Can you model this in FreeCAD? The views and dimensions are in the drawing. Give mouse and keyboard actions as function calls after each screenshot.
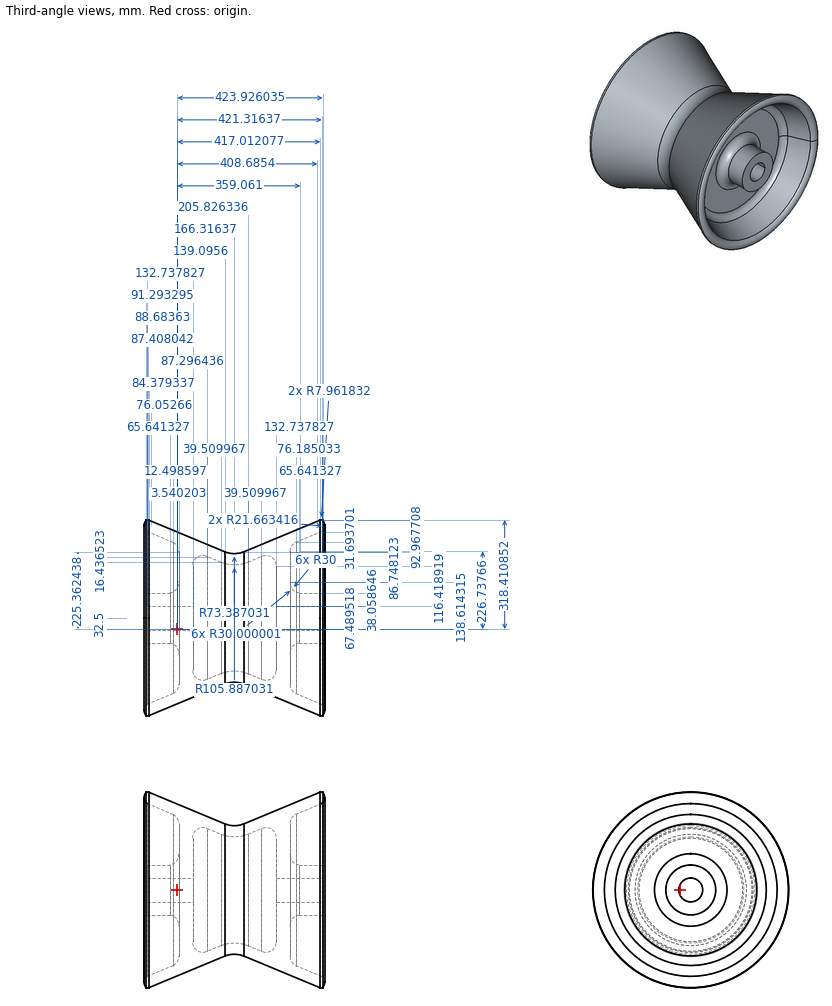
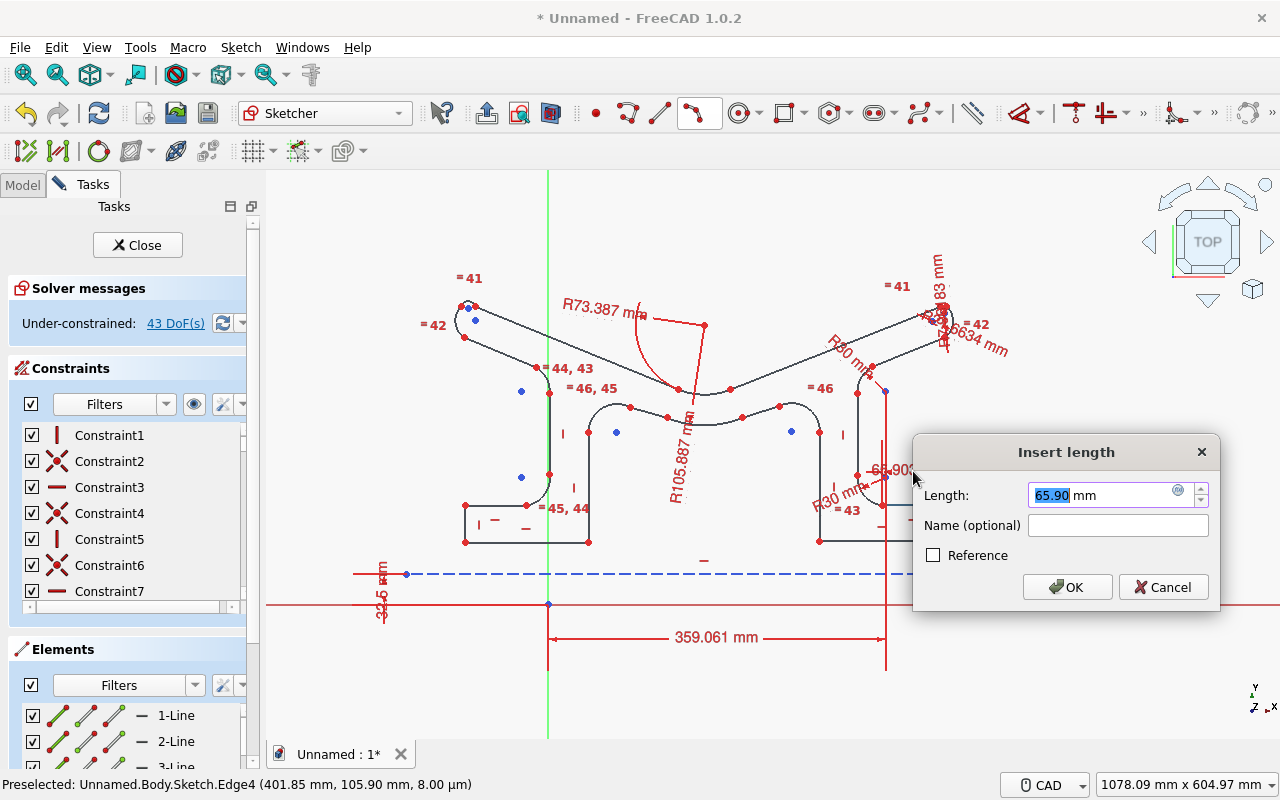
text(65.641327)
key(Return)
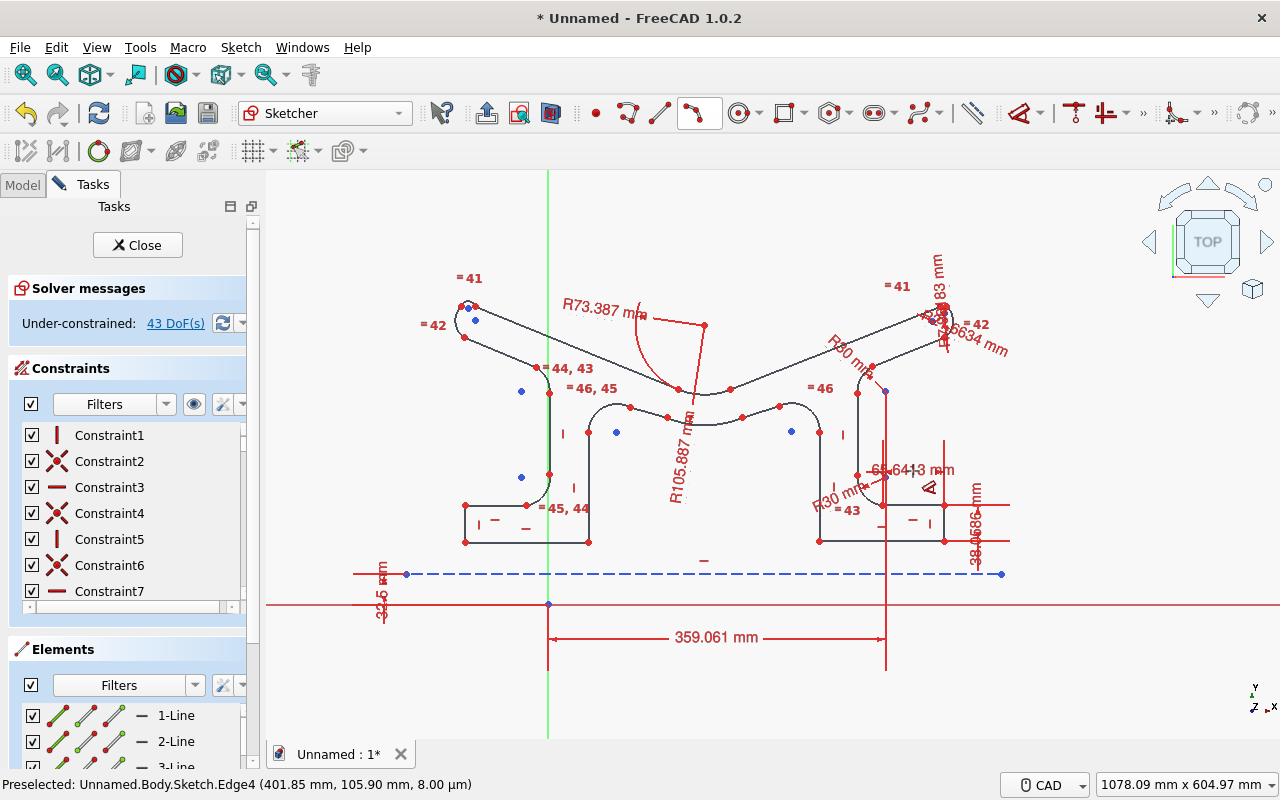
click(858, 451)
click(892, 435)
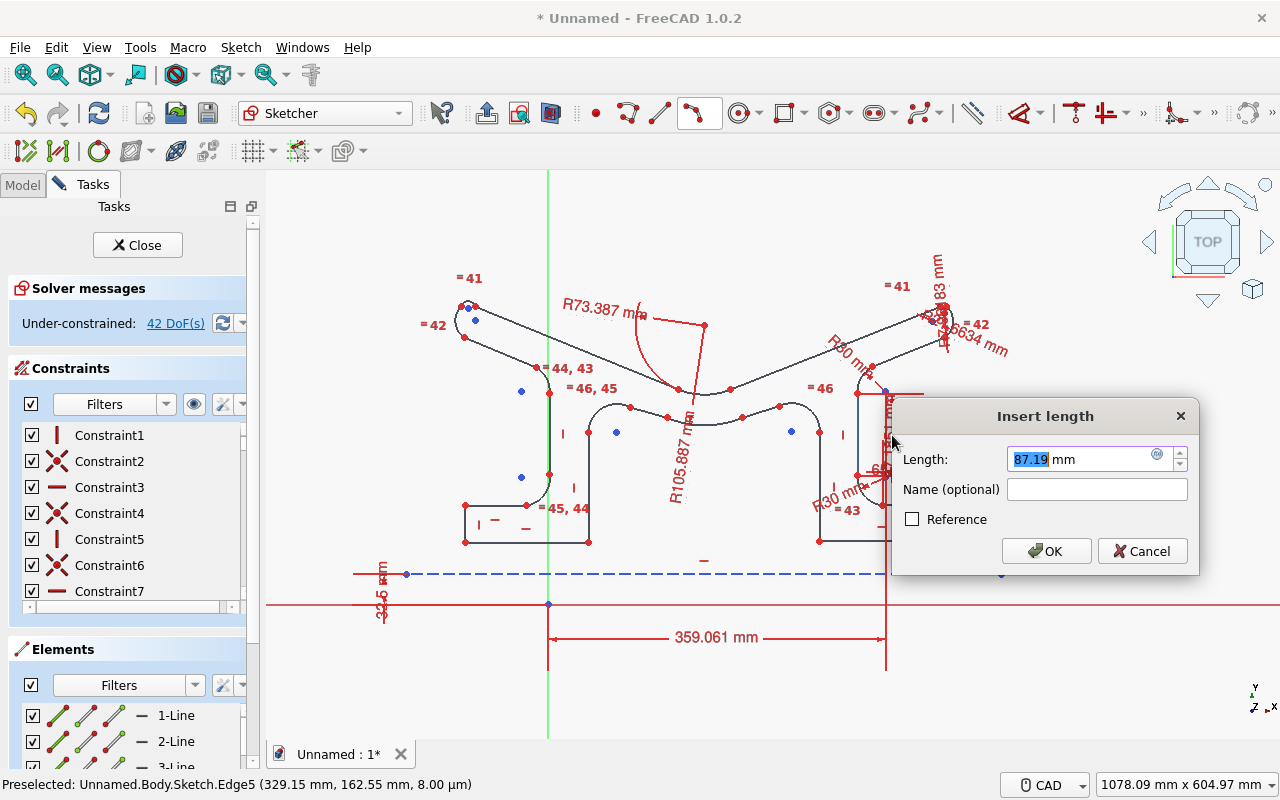
text(86.748123)
key(Return)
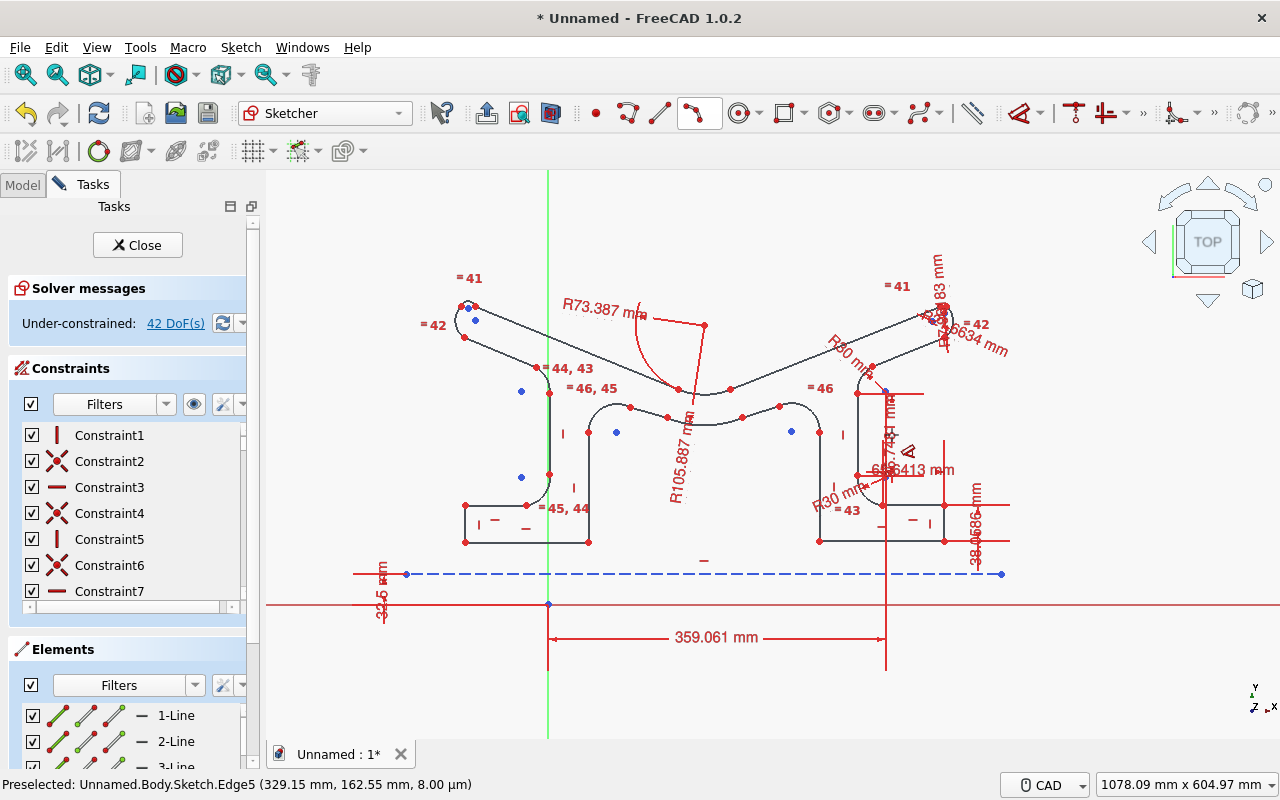
click(550, 418)
click(516, 434)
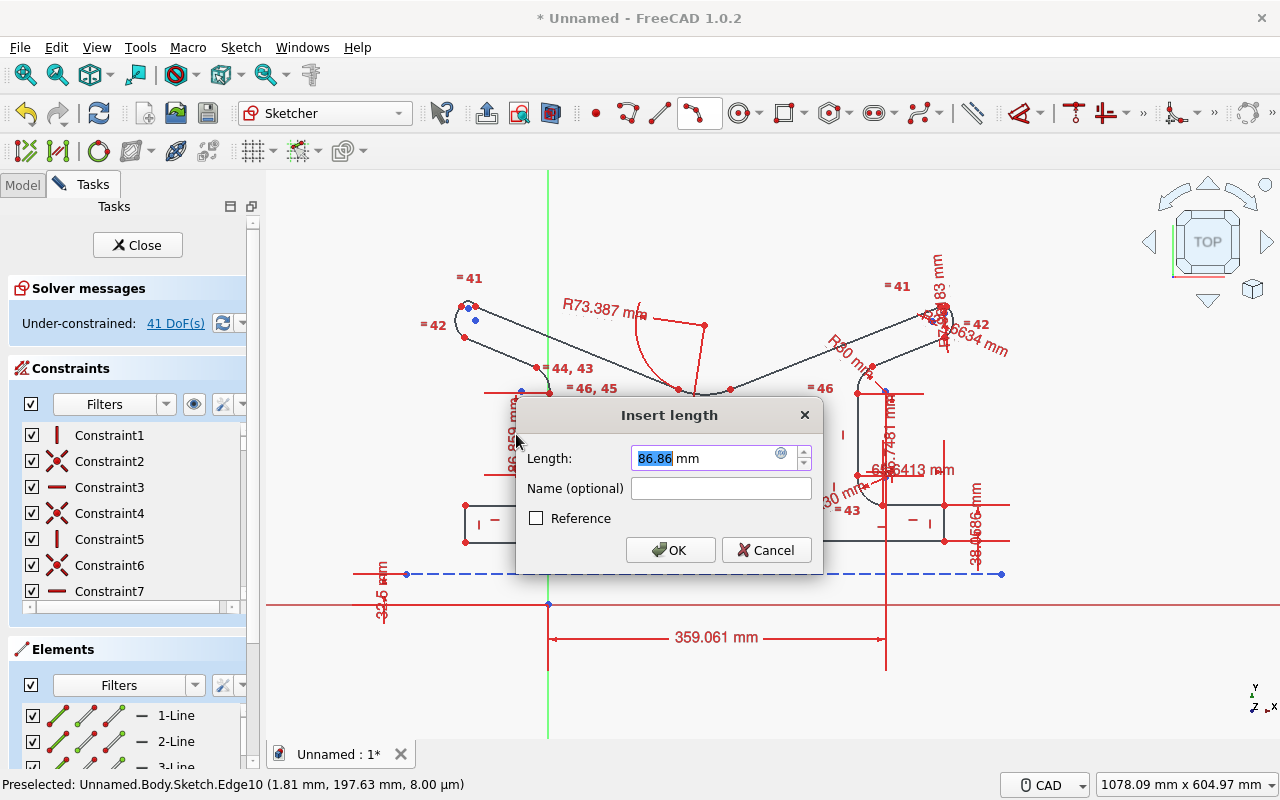
text(86.748123)
key(Return)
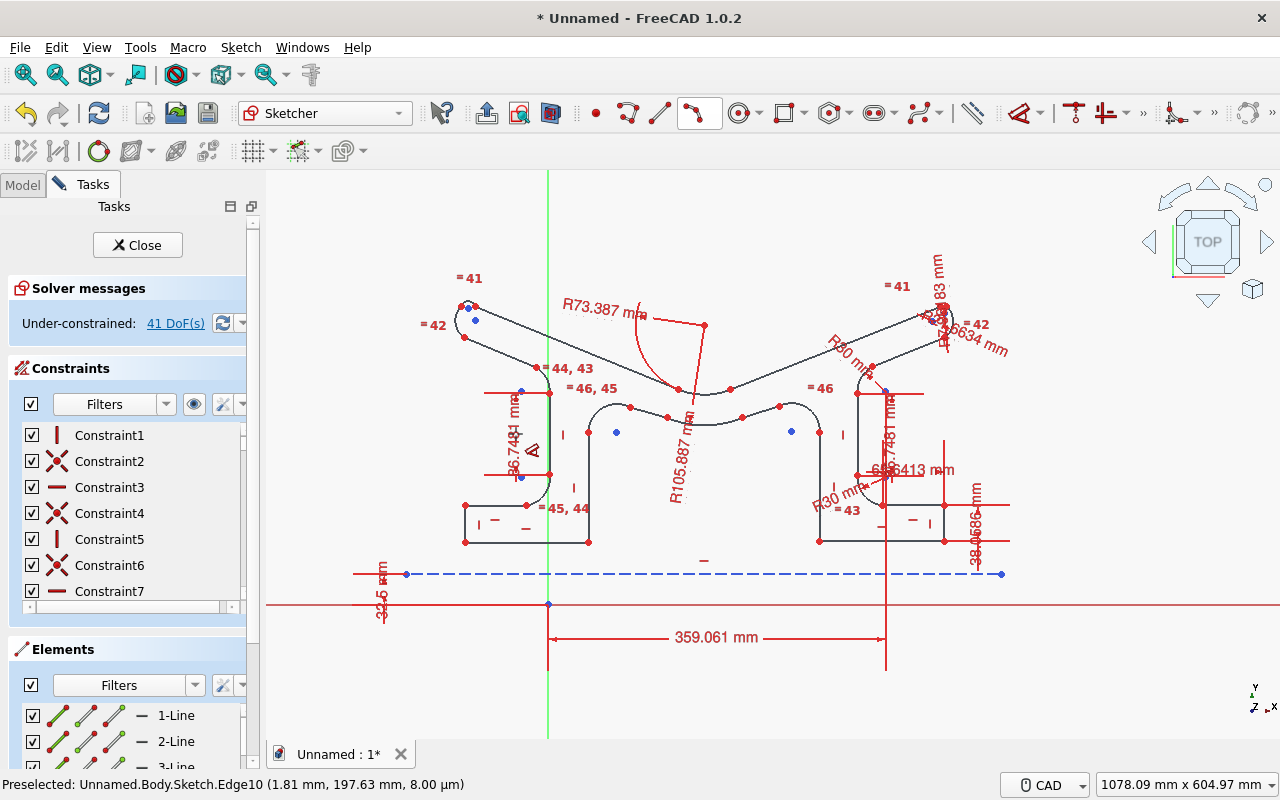
click(508, 506)
click(496, 472)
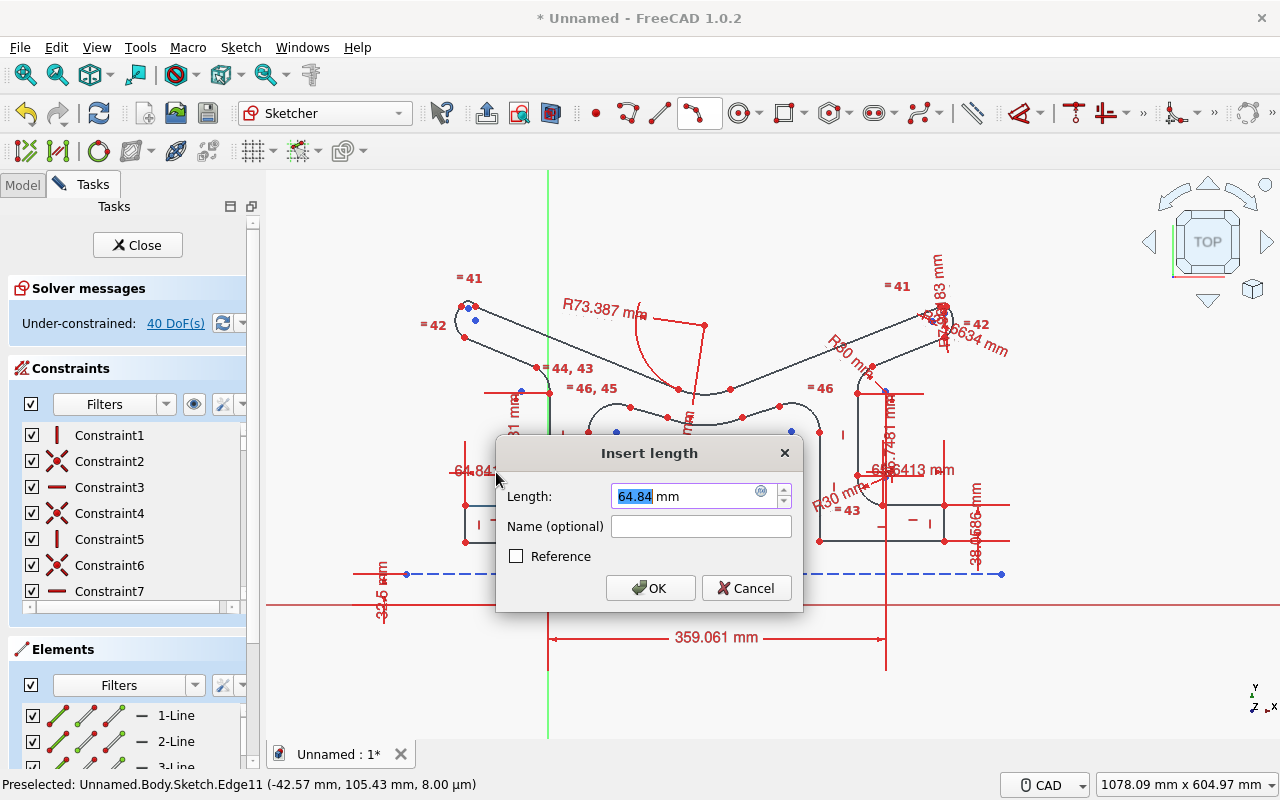
text(65.641327)
key(Return)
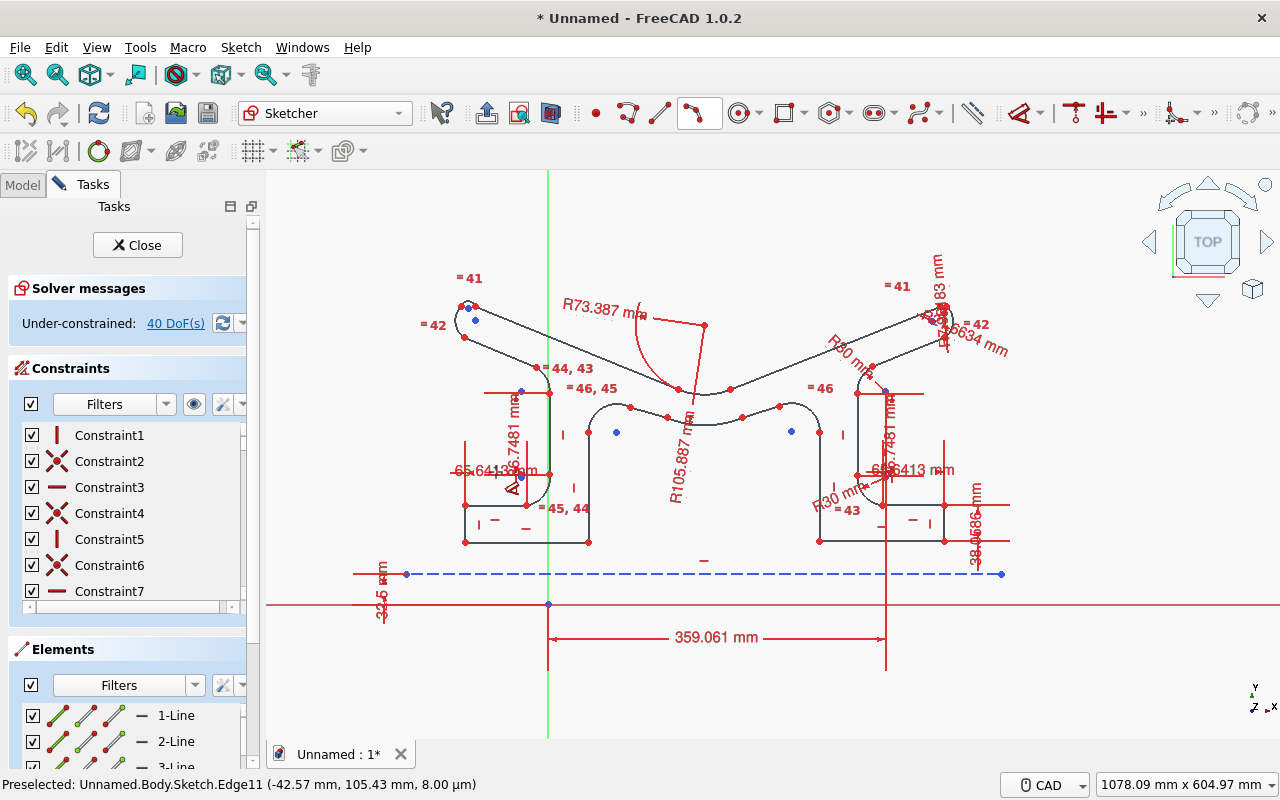
scroll(465, 517, up, 2)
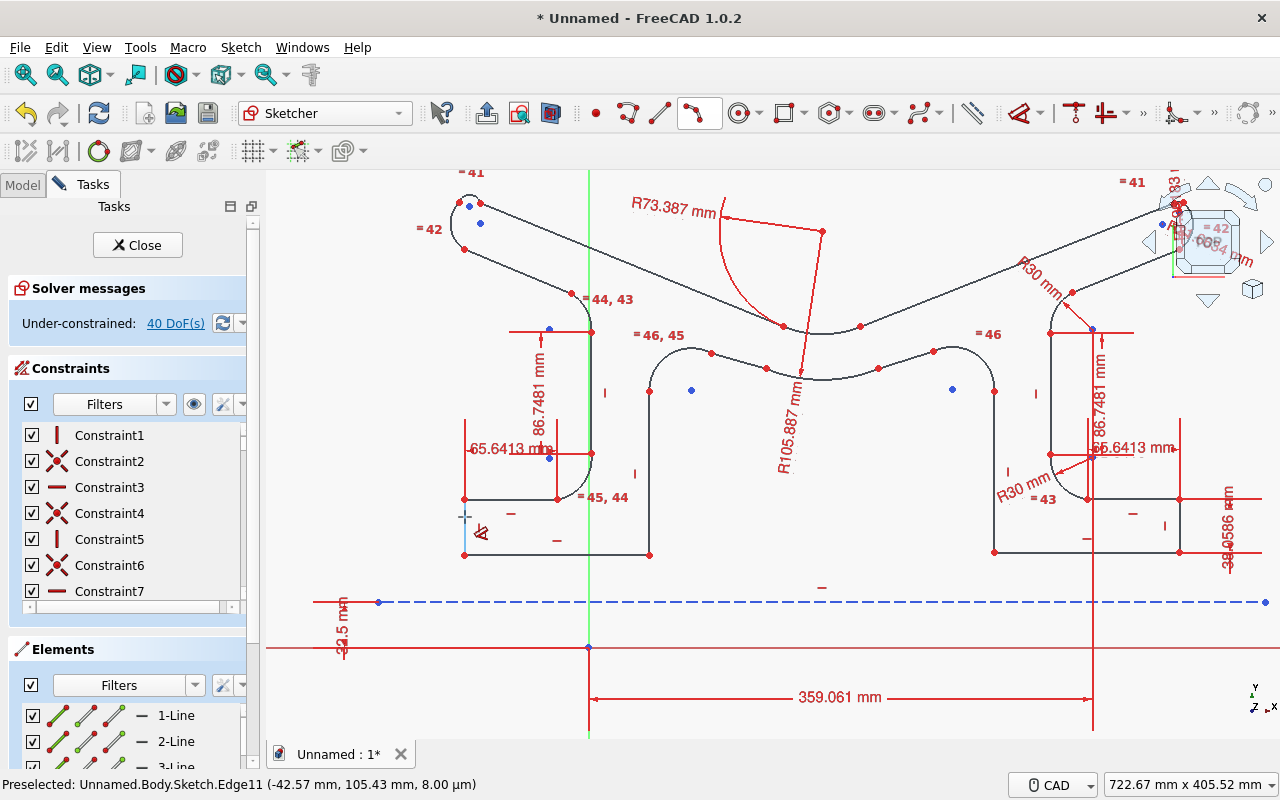
click(465, 516)
click(431, 527)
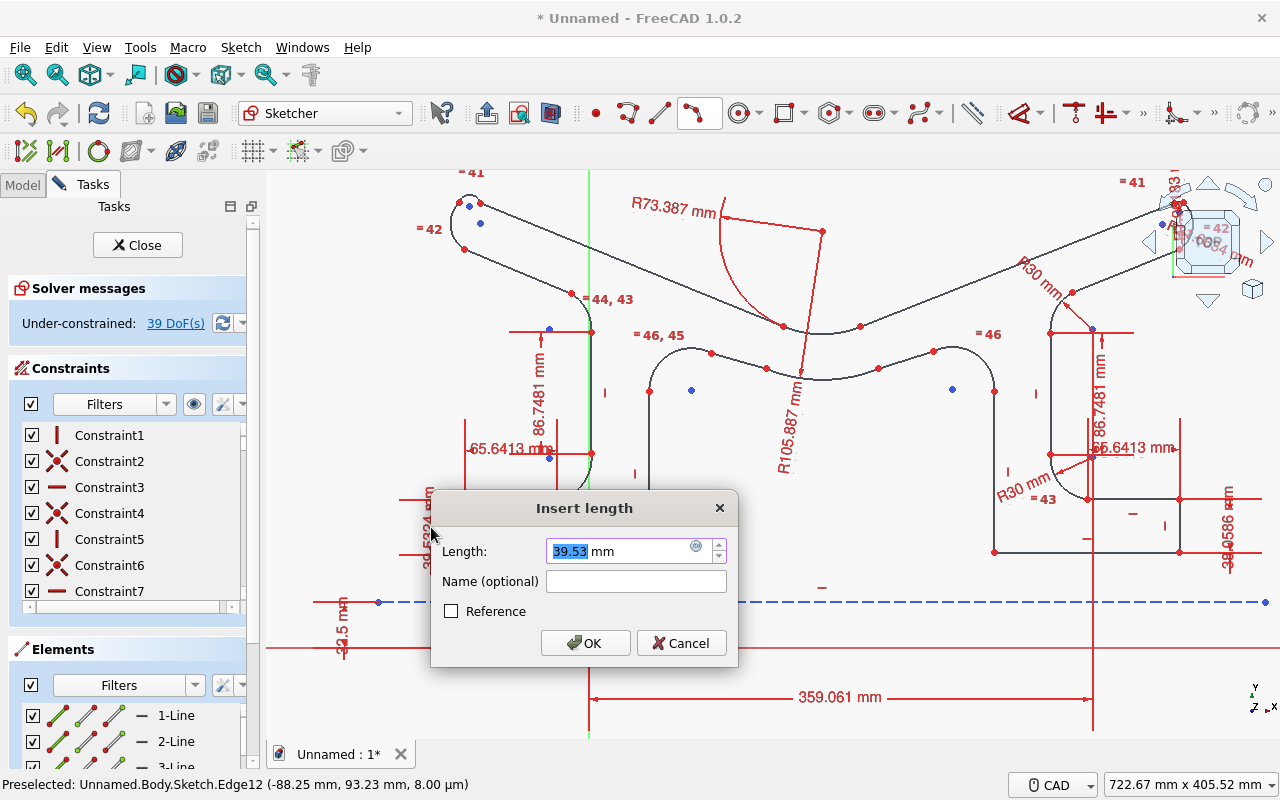
text(38.058646)
key(Return)